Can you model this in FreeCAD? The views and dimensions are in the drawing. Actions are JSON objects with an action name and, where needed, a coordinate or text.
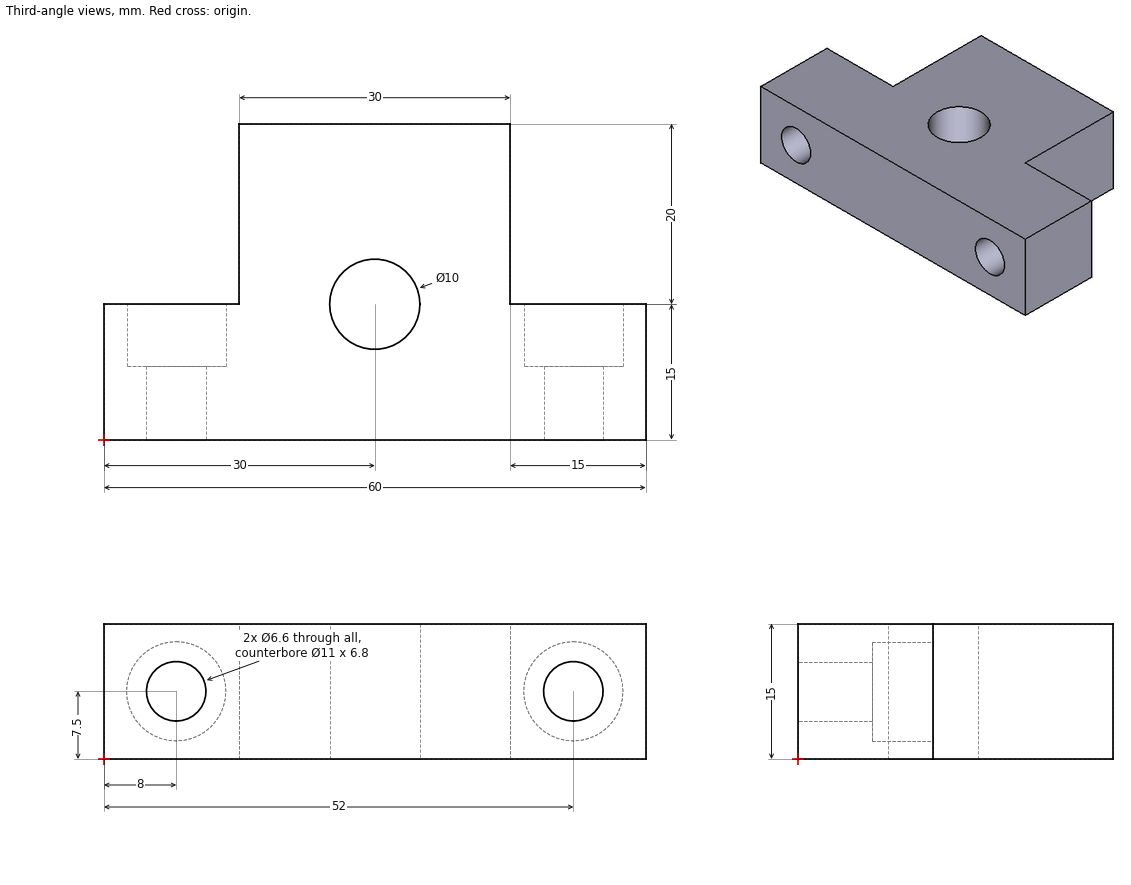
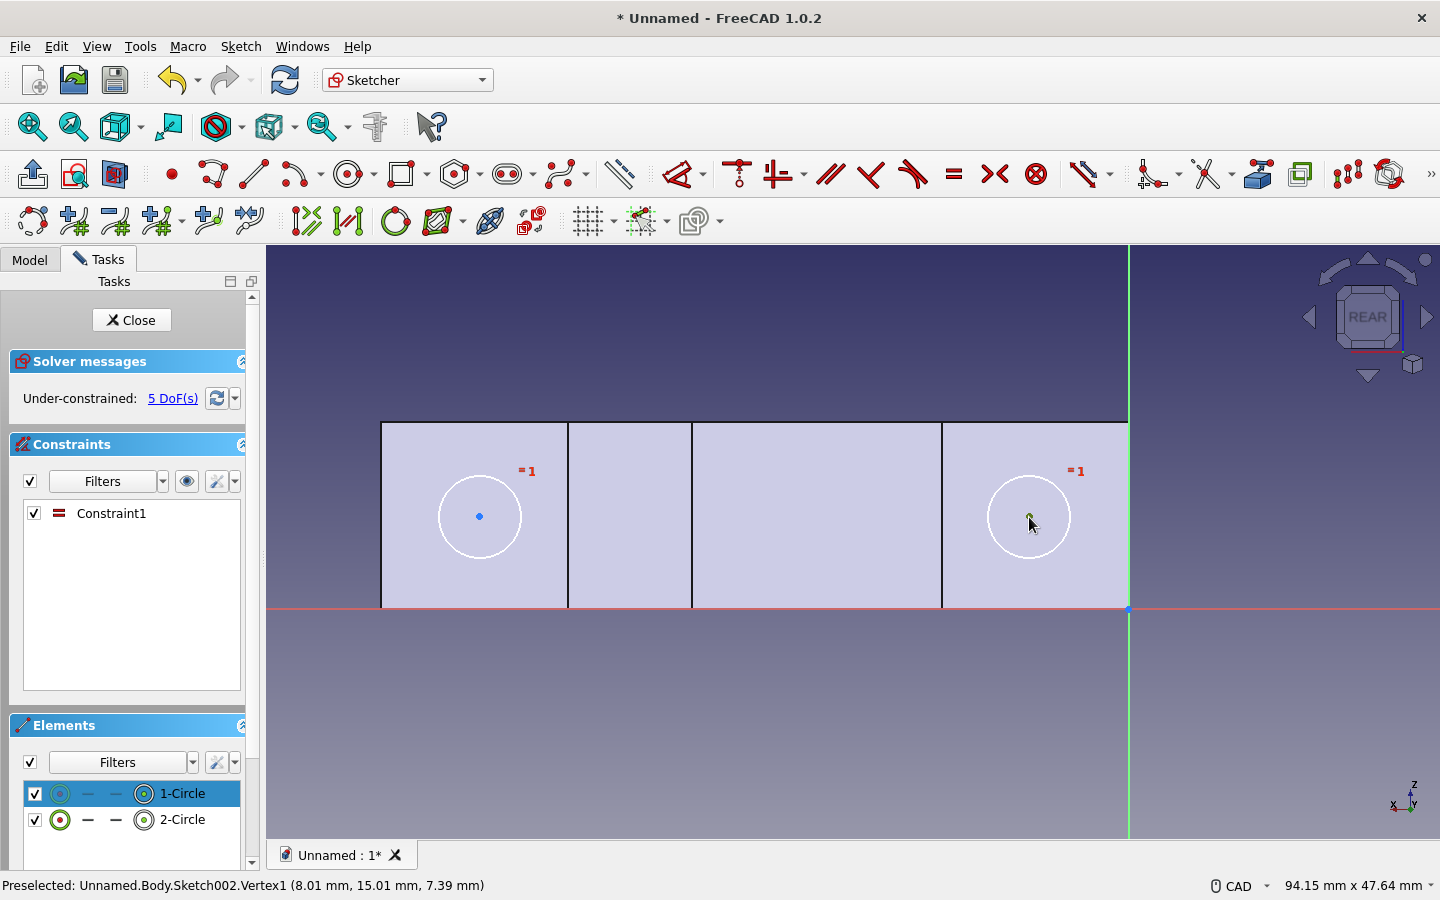
{"action": "left_click", "coordinate": [480, 517]}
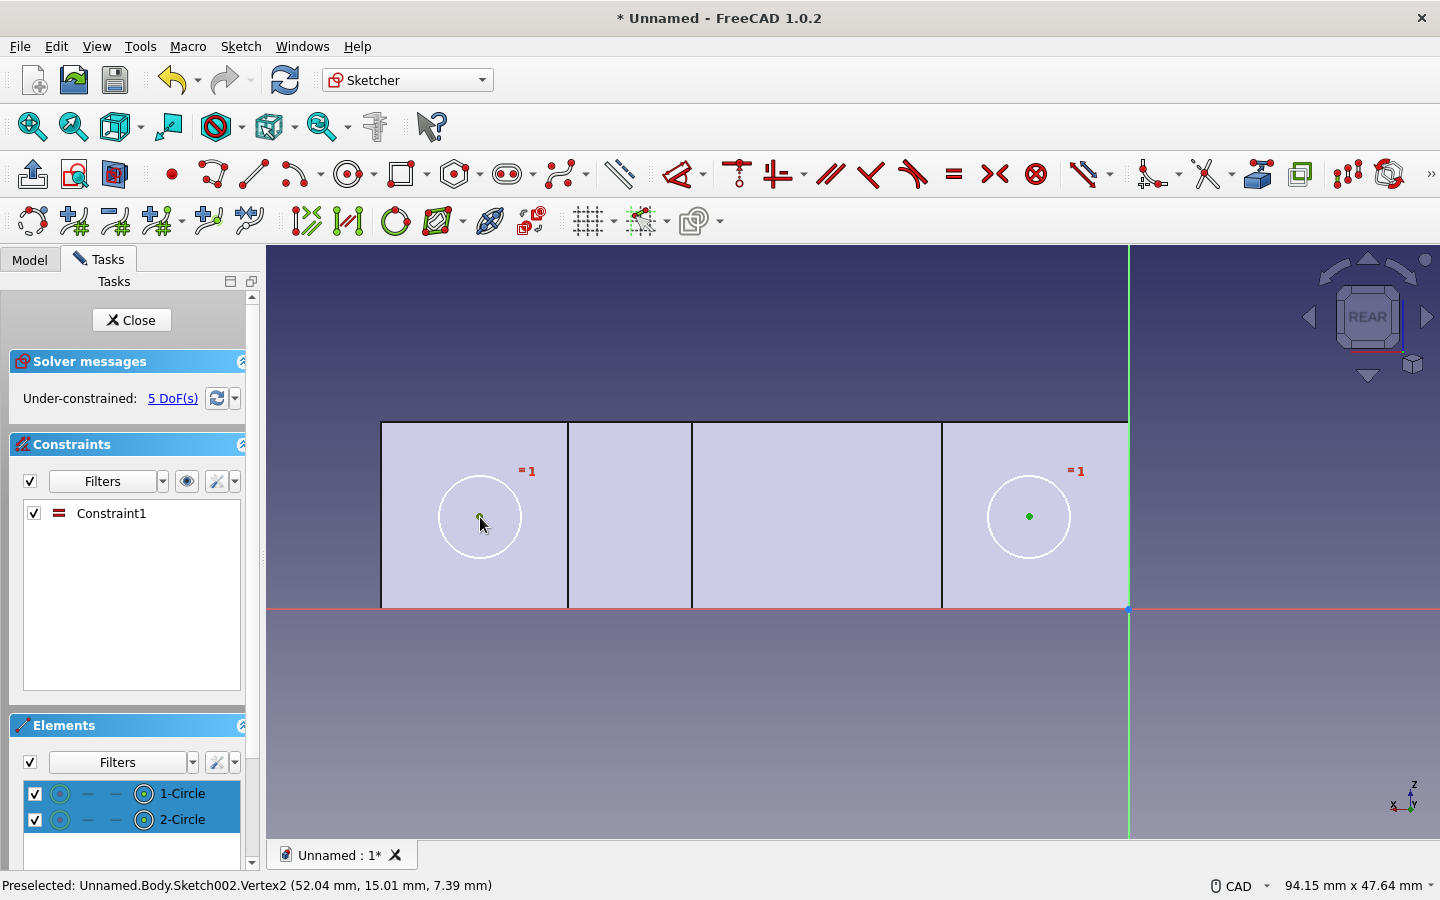
{"action": "left_click", "coordinate": [804, 174]}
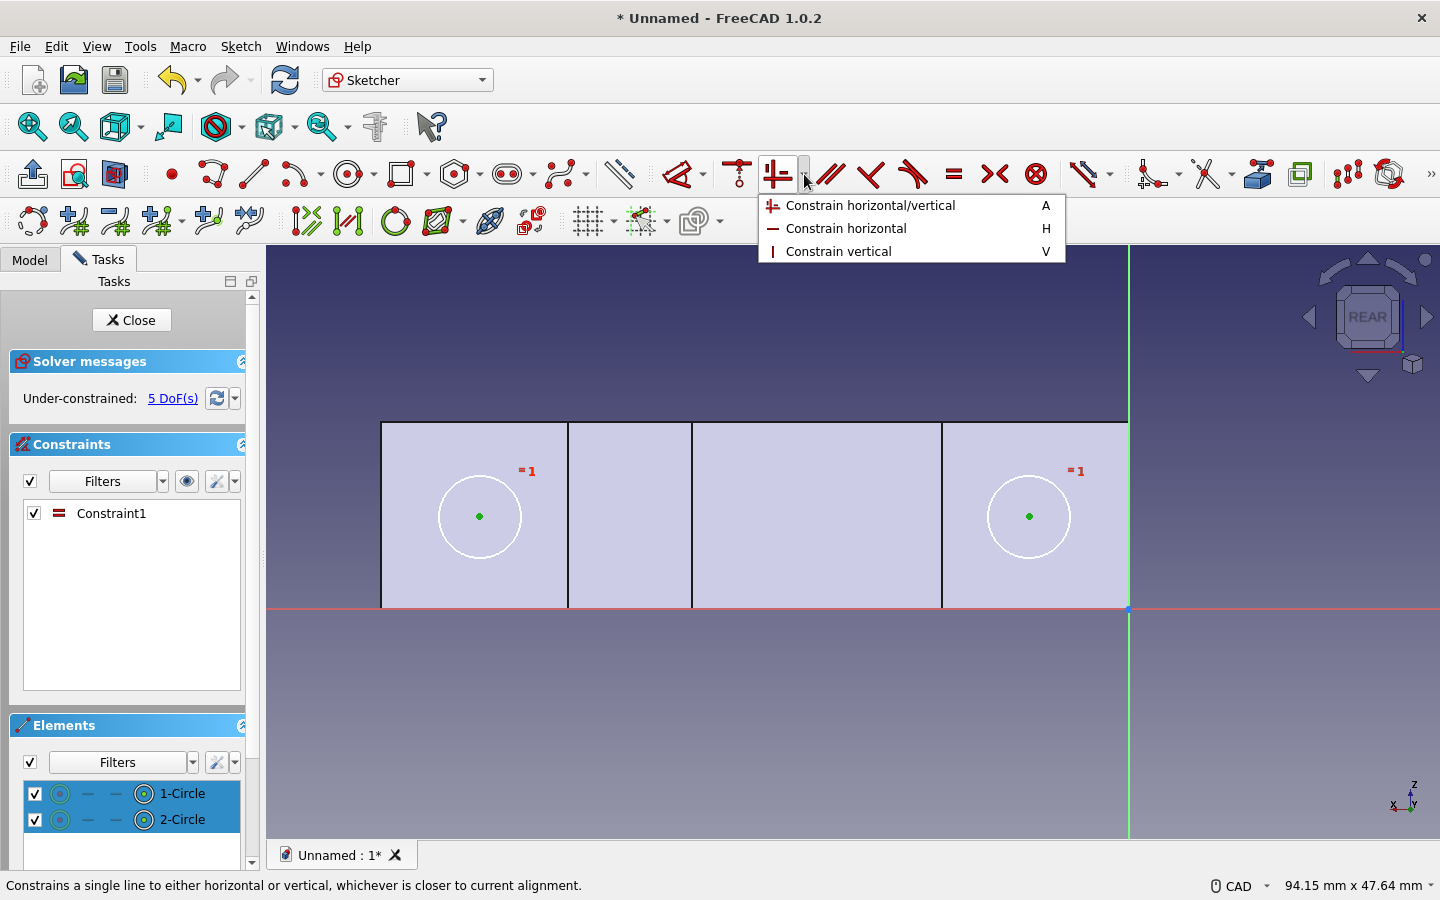
{"action": "left_click", "coordinate": [912, 228]}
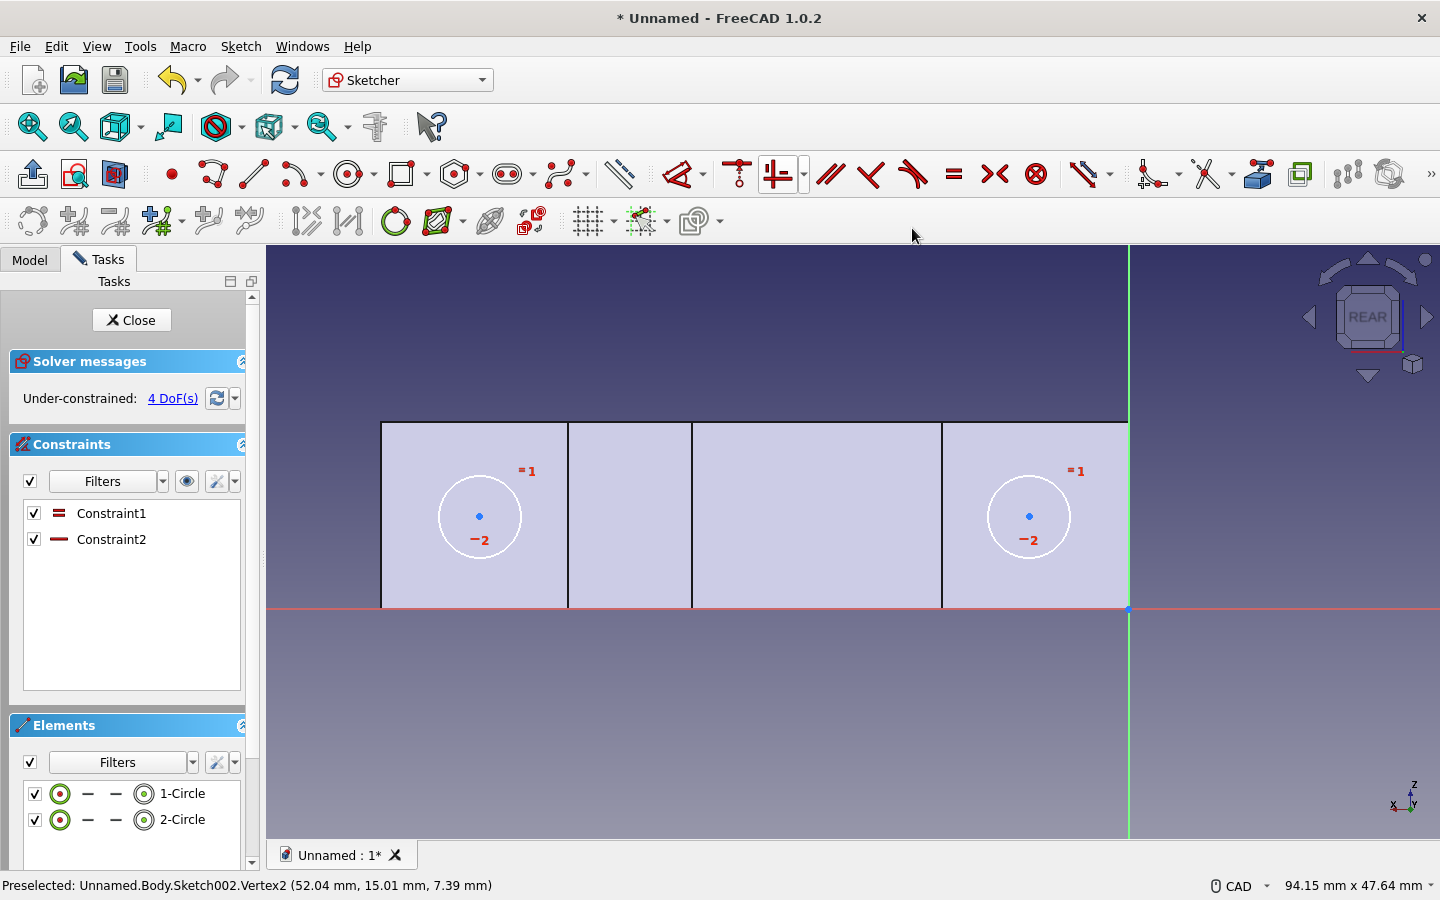
{"action": "left_click", "coordinate": [676, 174]}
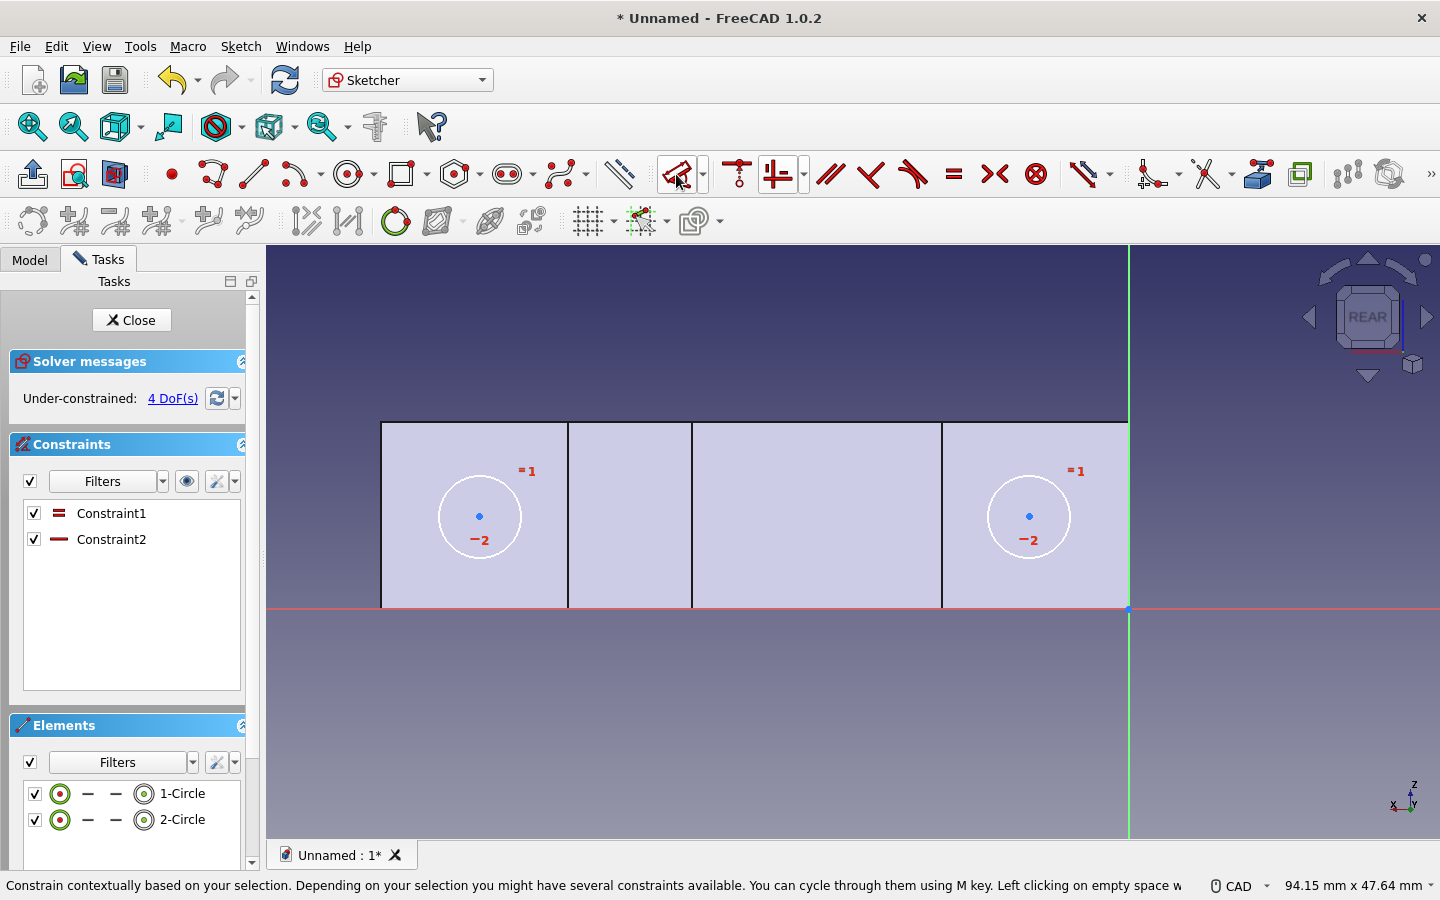
{"action": "left_click", "coordinate": [1058, 488]}
{"action": "left_click", "coordinate": [1081, 465]}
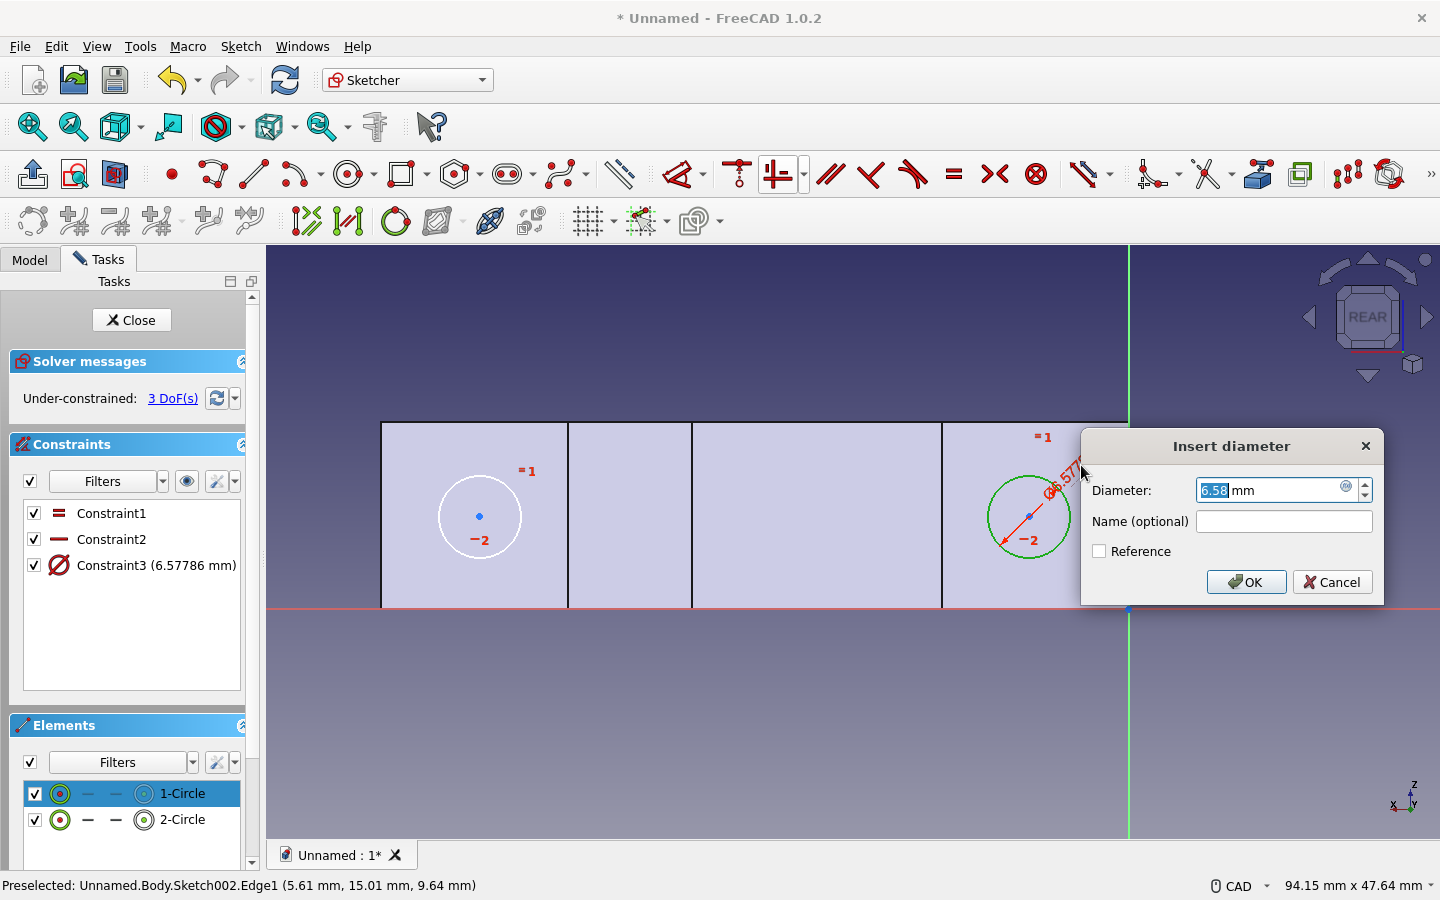
{"action": "type", "text": "6.6"}
{"action": "key", "text": "Return"}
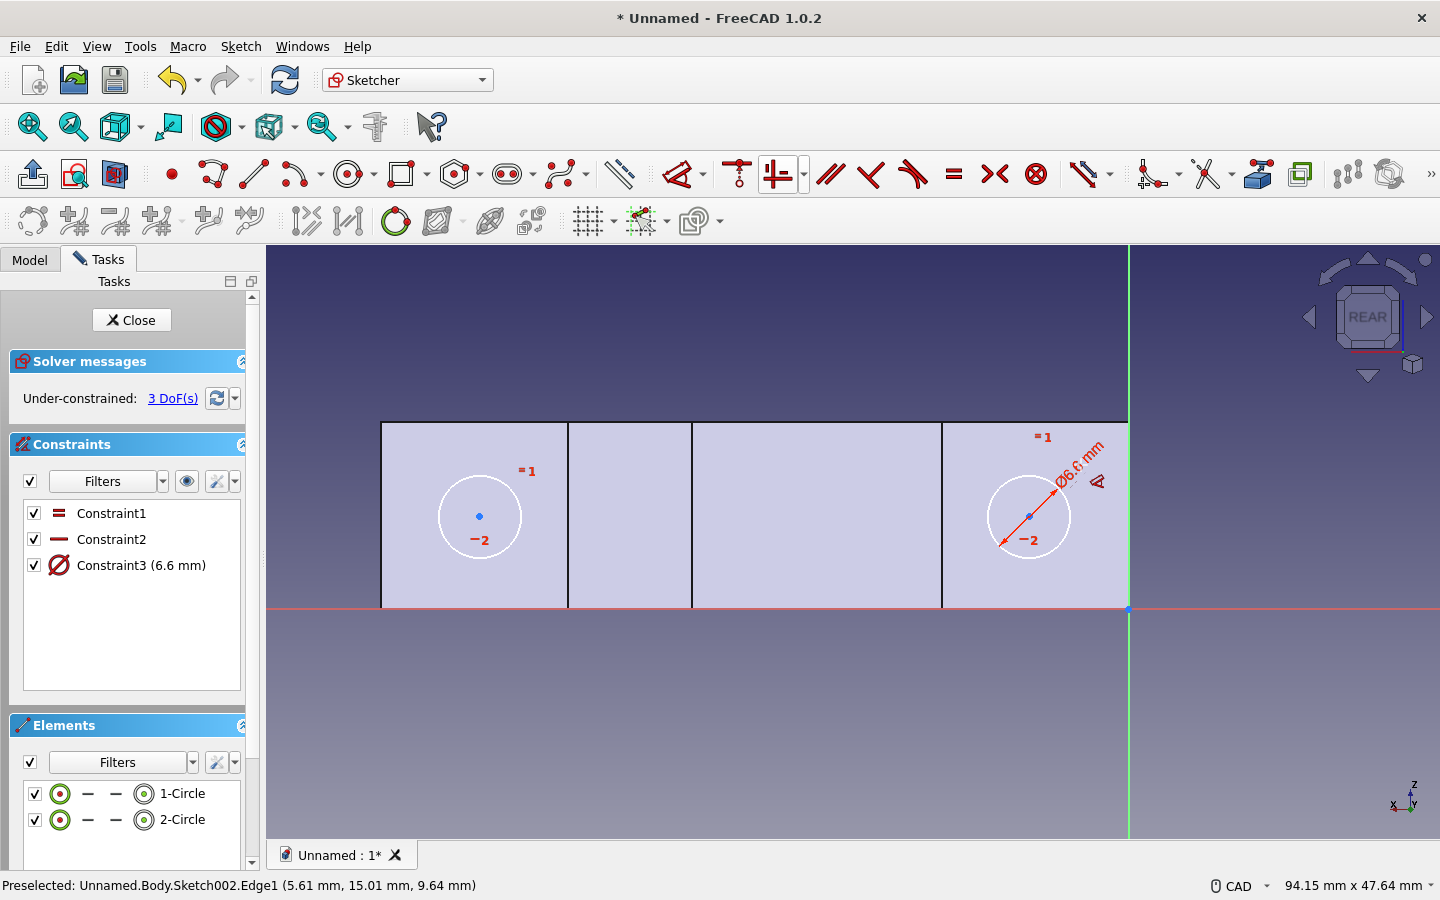
{"action": "left_click", "coordinate": [1029, 517]}
{"action": "left_click", "coordinate": [1079, 643]}